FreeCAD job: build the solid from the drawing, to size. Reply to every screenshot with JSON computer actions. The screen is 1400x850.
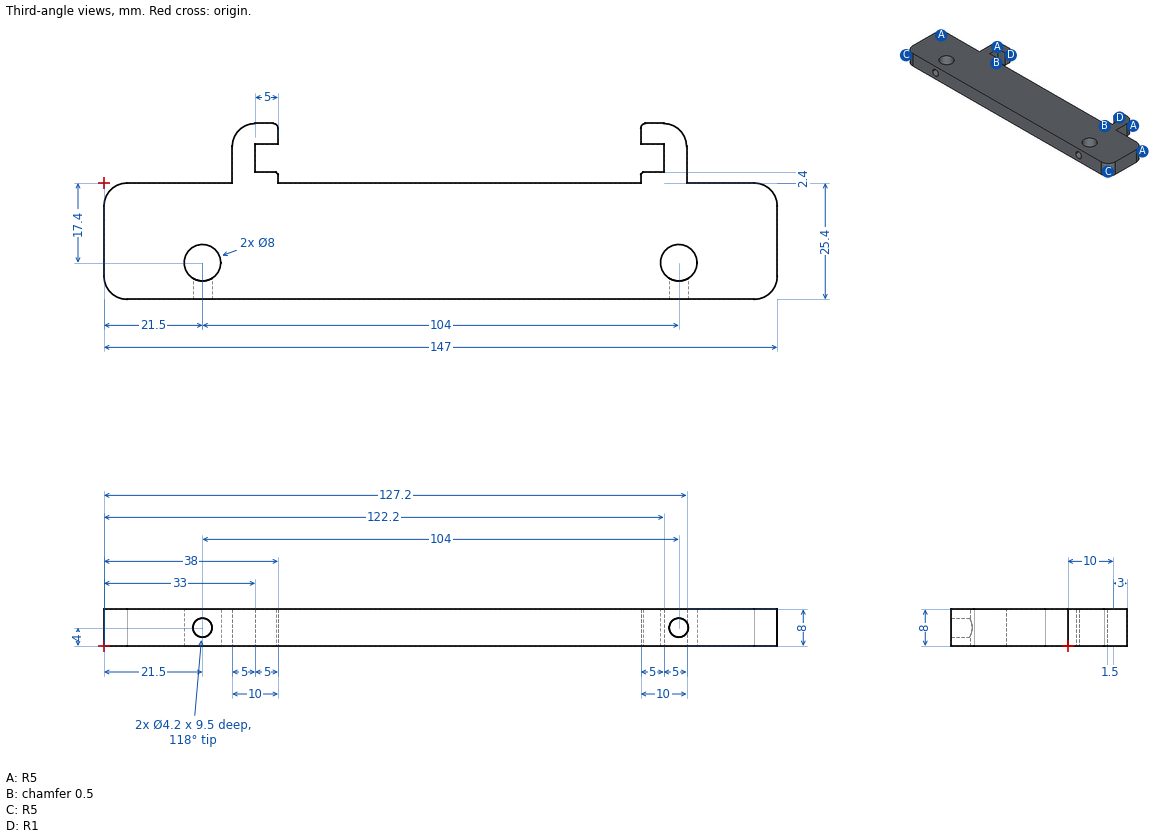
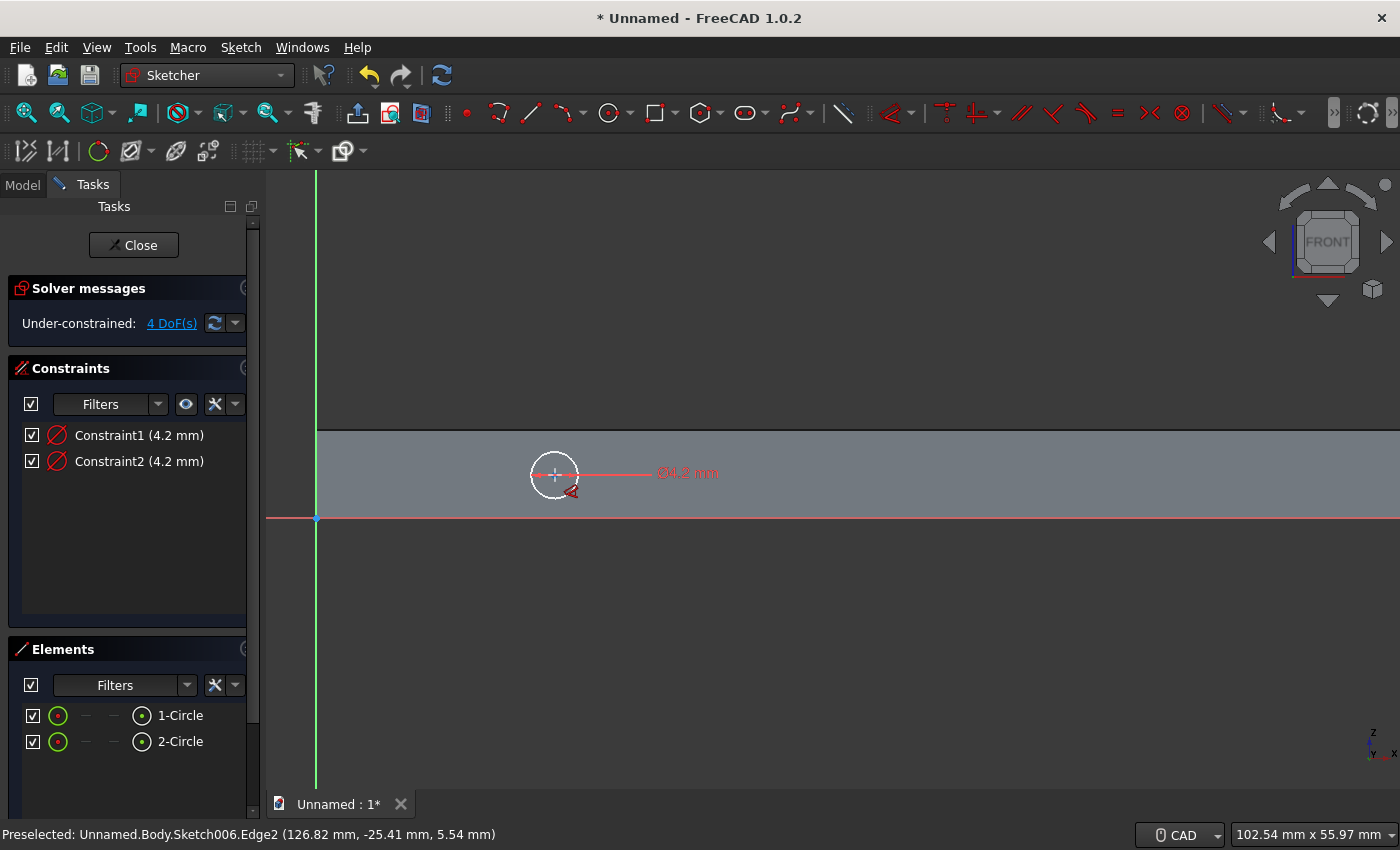
{"action": "left_click", "coordinate": [555, 475]}
{"action": "left_click", "coordinate": [589, 497]}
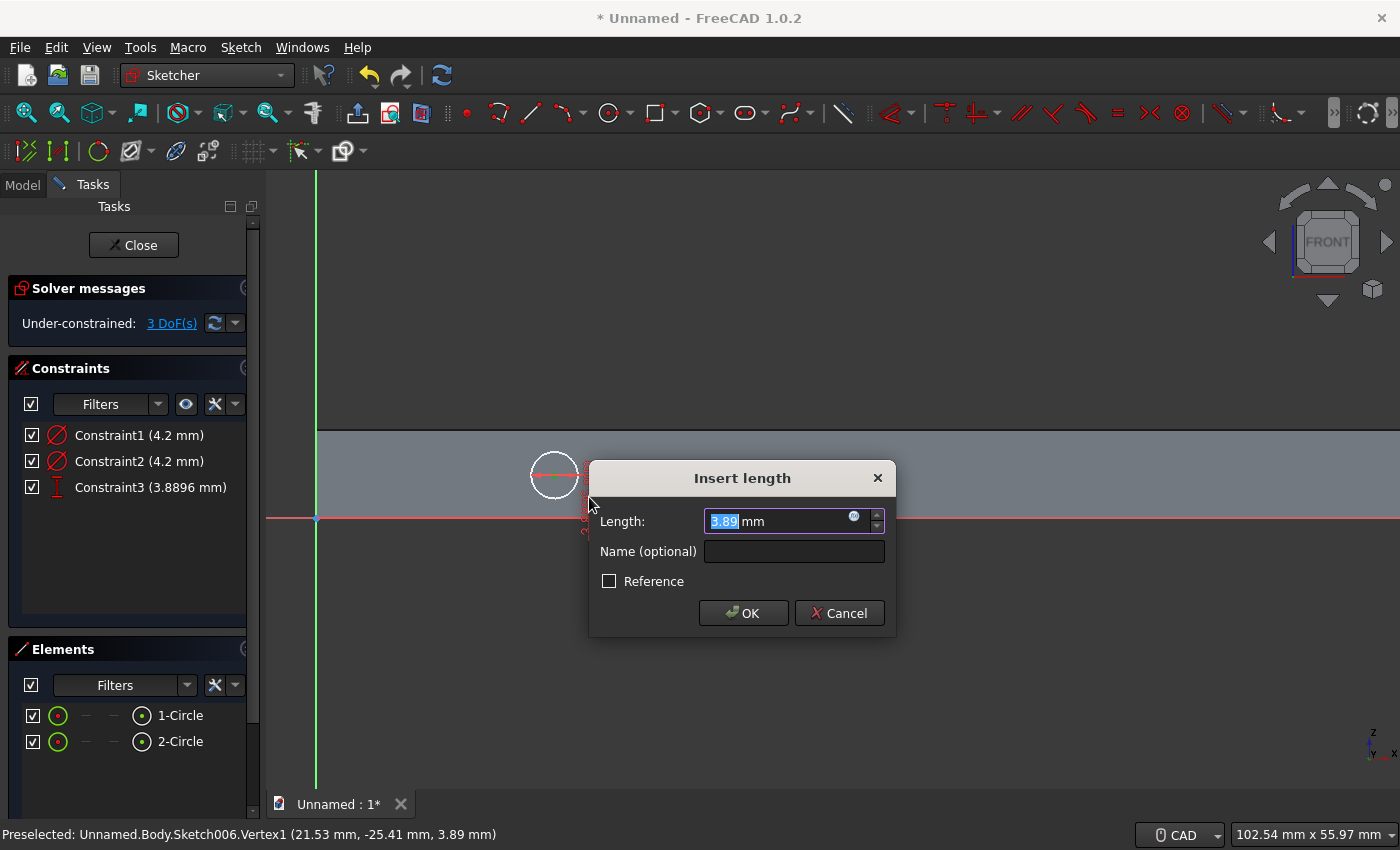
{"action": "type", "text": "4"}
{"action": "key", "text": "Return"}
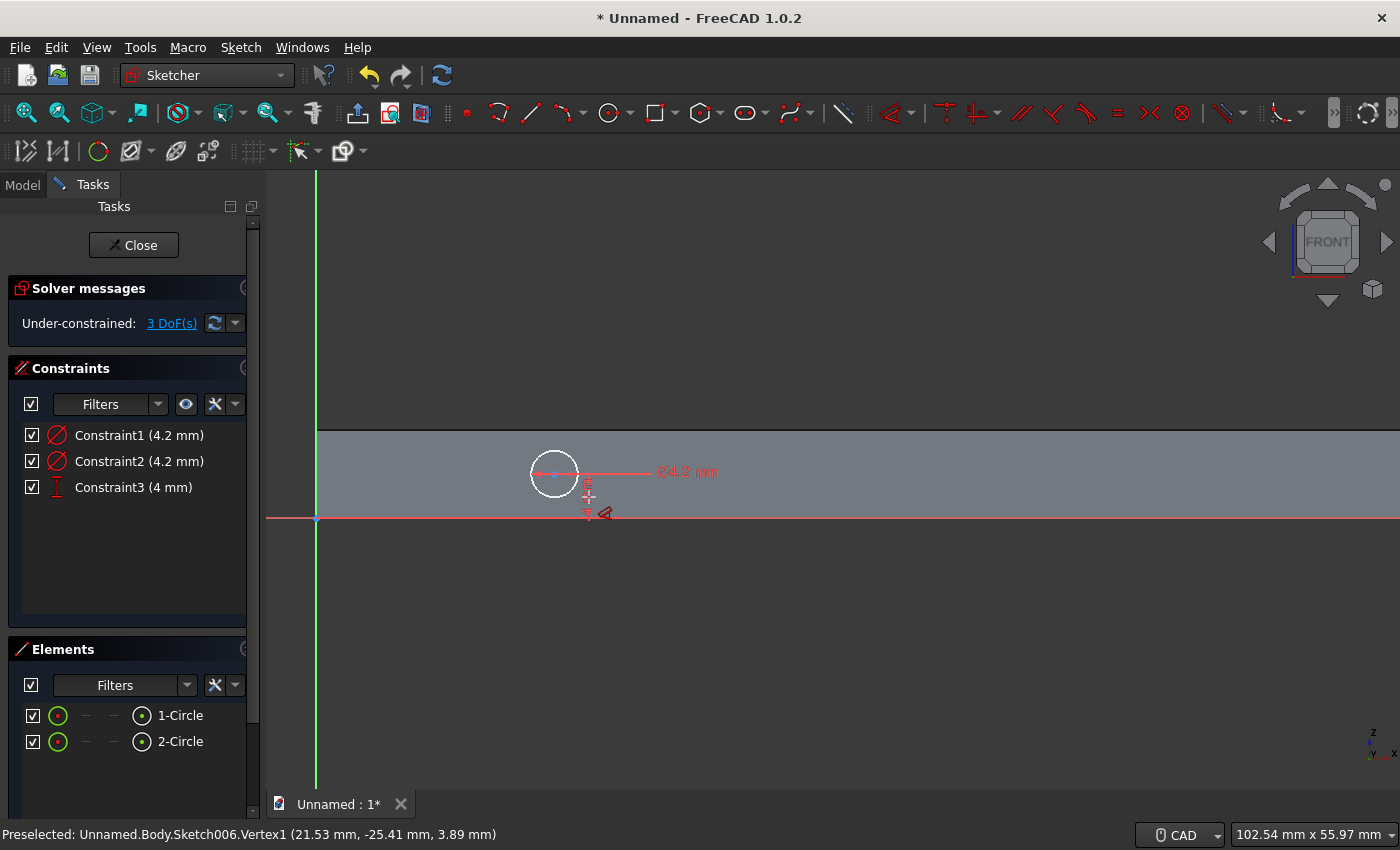
{"action": "scroll", "coordinate": [554, 475], "scroll_direction": "down", "scroll_amount": 4}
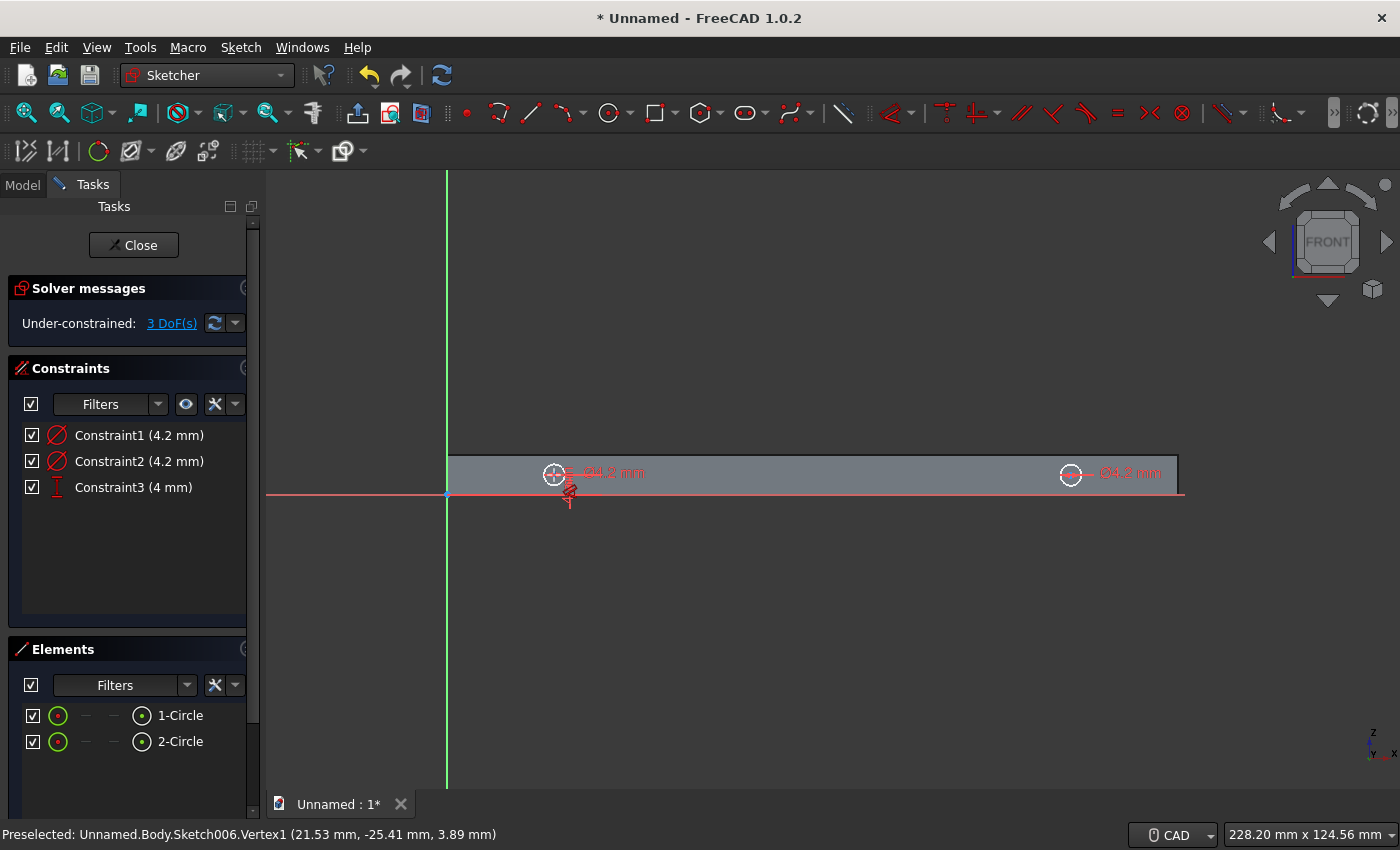
{"action": "scroll", "coordinate": [1071, 475], "scroll_direction": "up", "scroll_amount": 4}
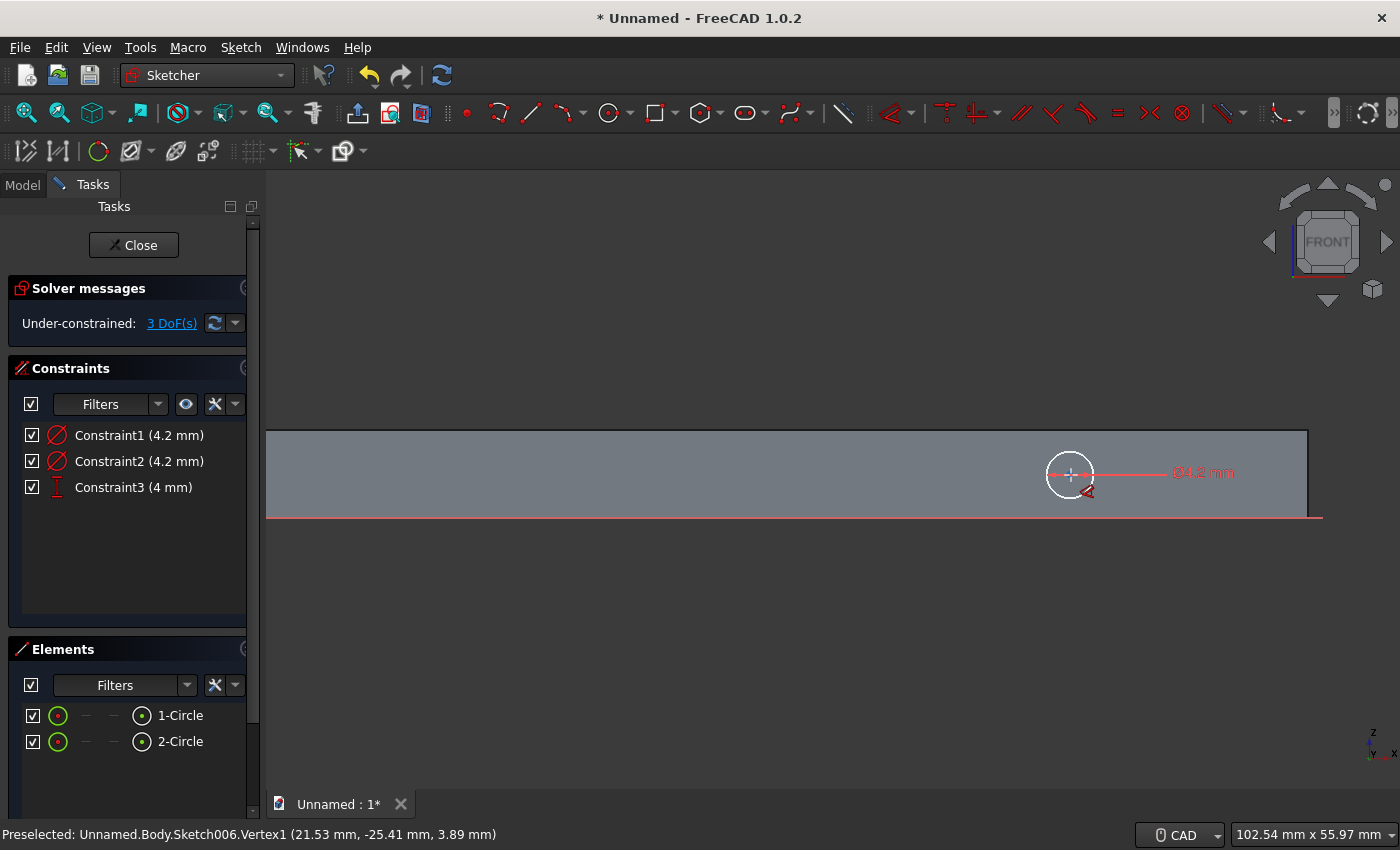
{"action": "left_click", "coordinate": [1070, 475]}
{"action": "left_click", "coordinate": [1104, 497]}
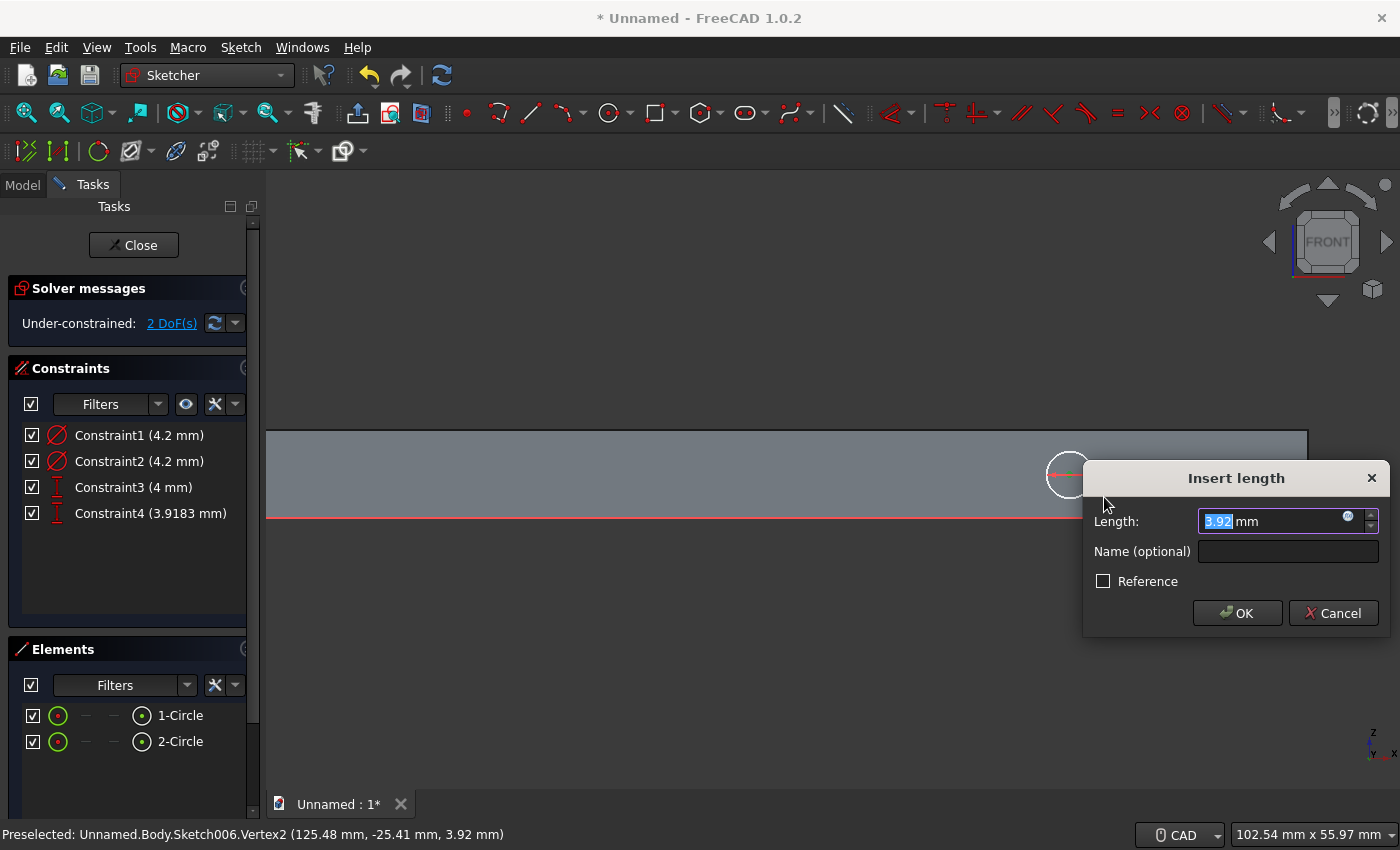
{"action": "type", "text": "4"}
{"action": "key", "text": "Return"}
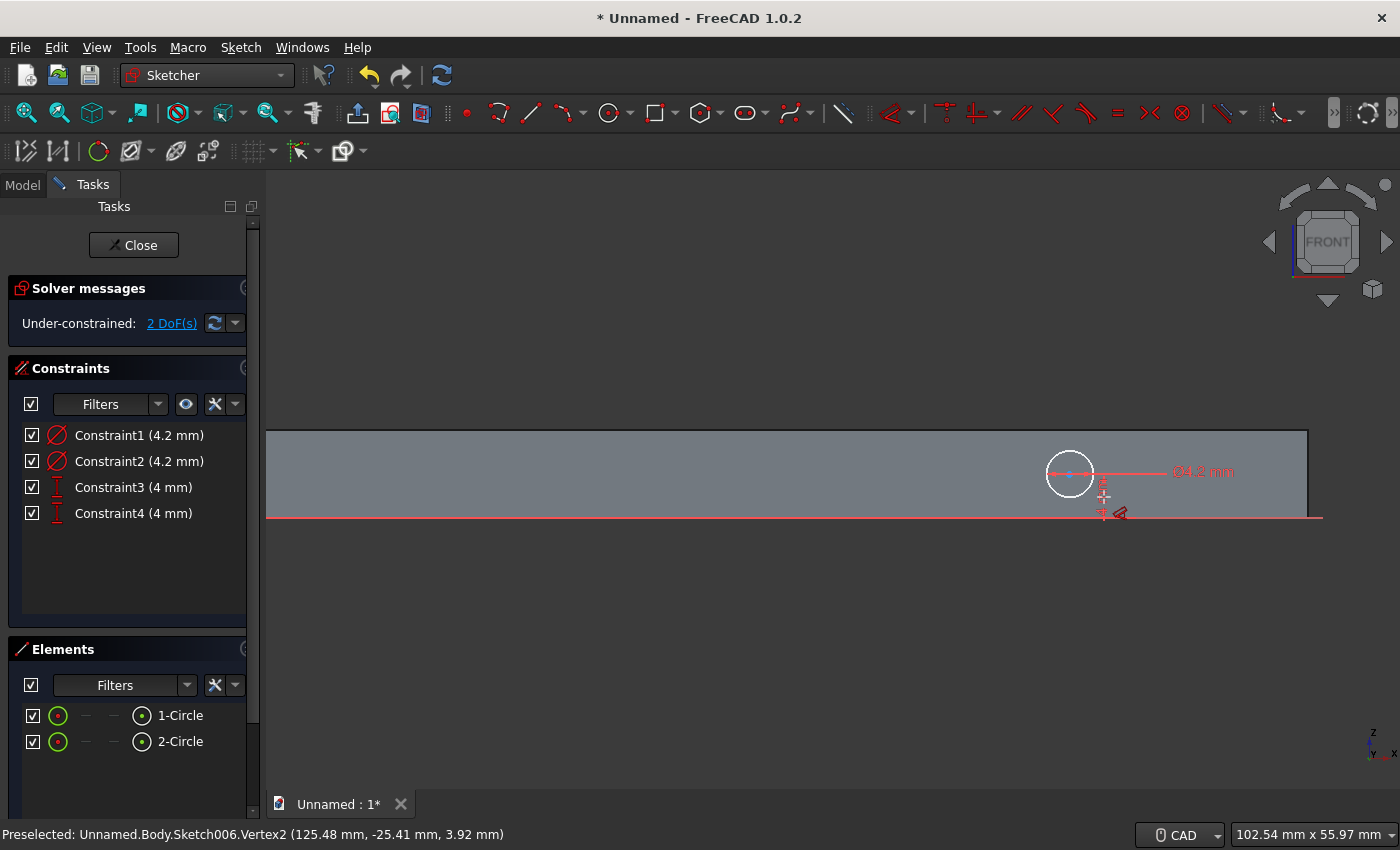
{"action": "scroll", "coordinate": [1072, 475], "scroll_direction": "down", "scroll_amount": 4}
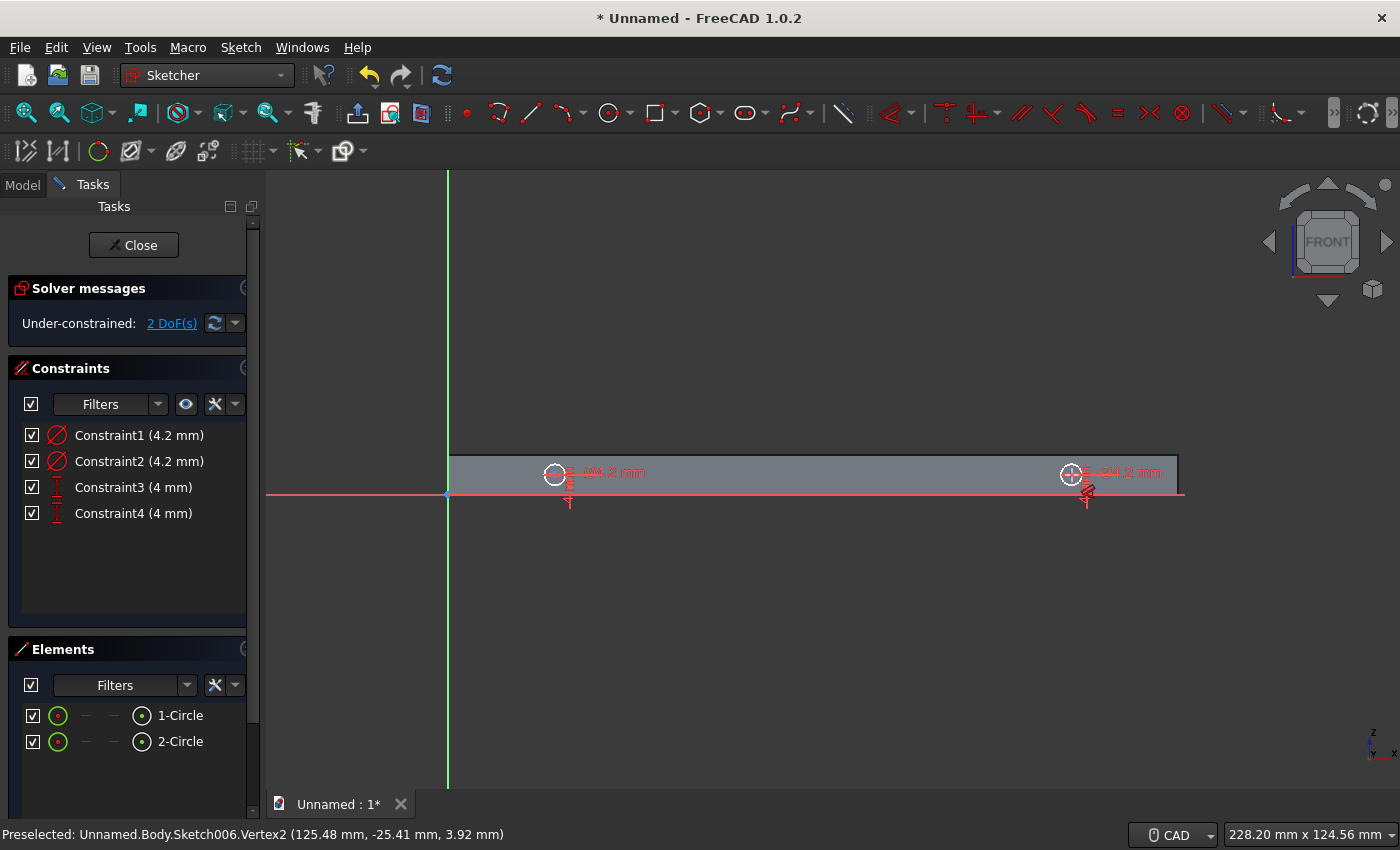
{"action": "left_click", "coordinate": [555, 475]}
{"action": "left_click", "coordinate": [501, 529]}